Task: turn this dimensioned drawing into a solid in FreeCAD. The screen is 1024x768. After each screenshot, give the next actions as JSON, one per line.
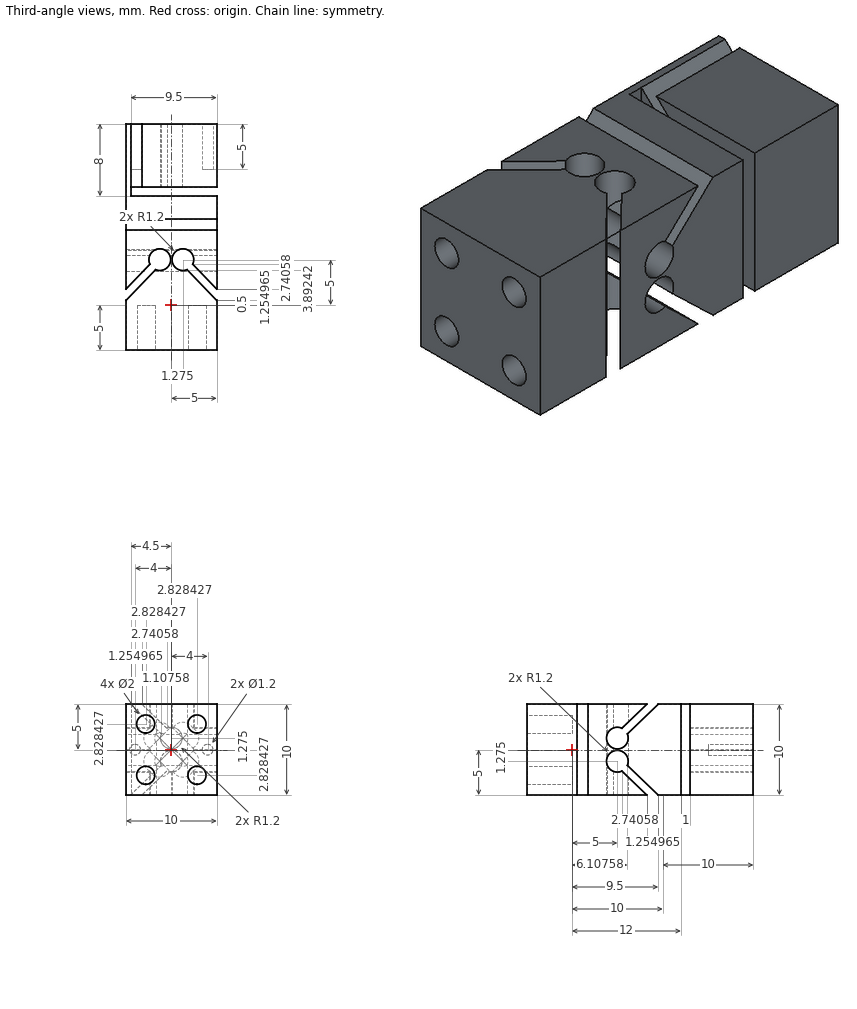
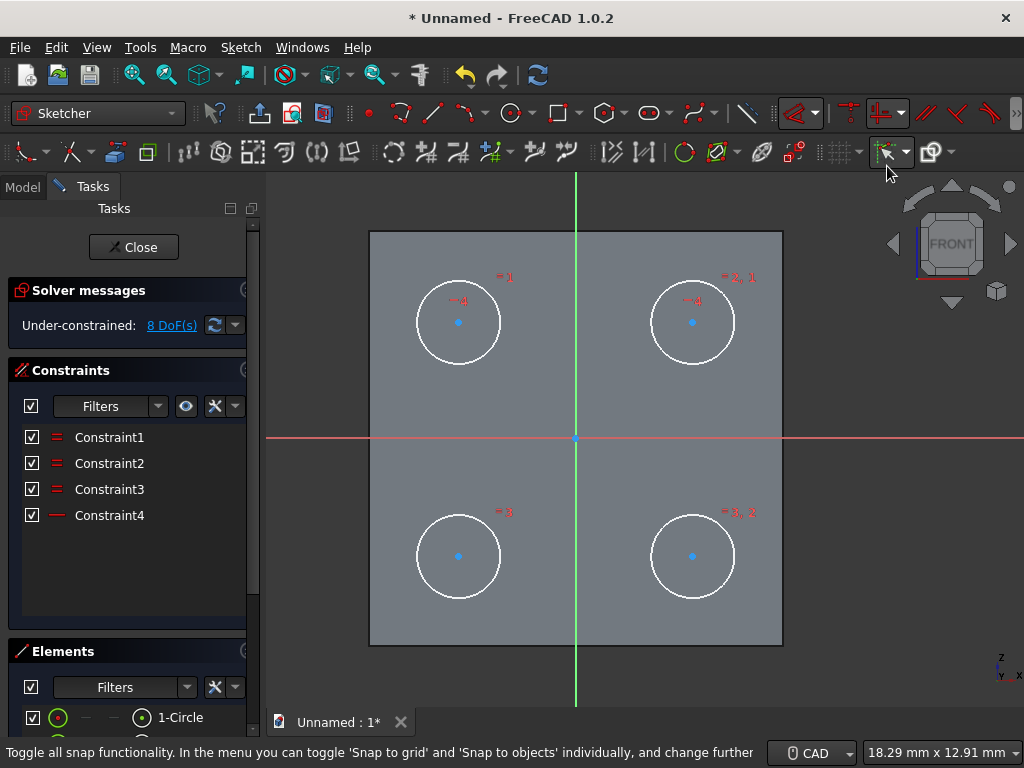
{"action": "left_click", "coordinate": [693, 322]}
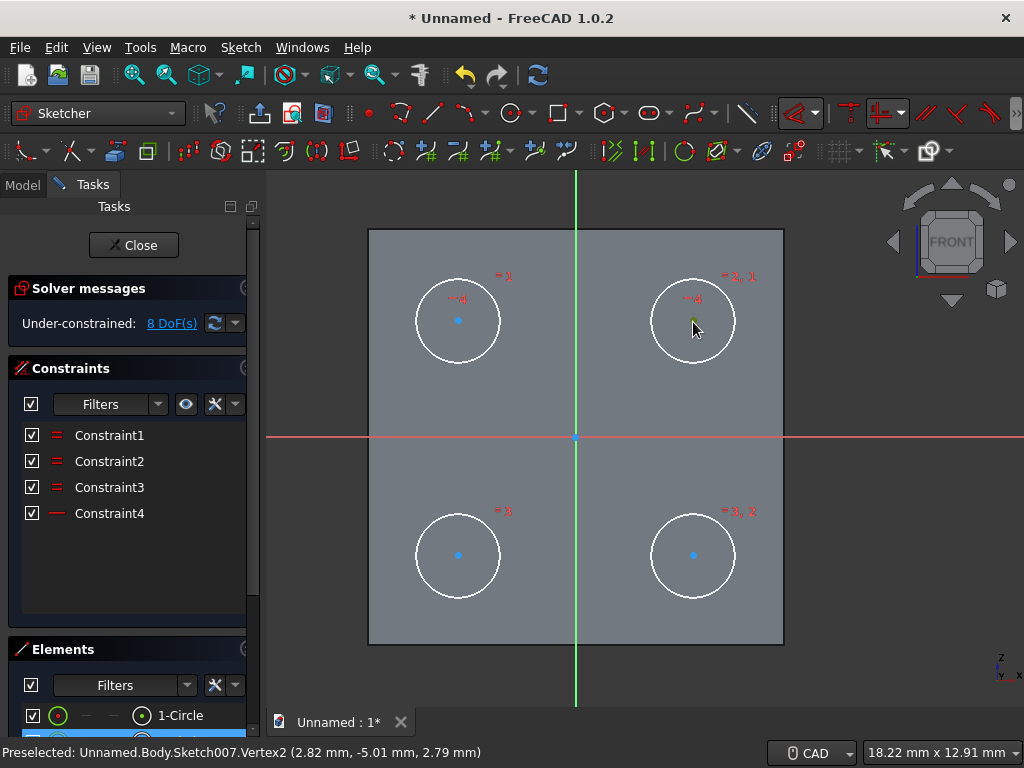
{"action": "left_click", "coordinate": [693, 556]}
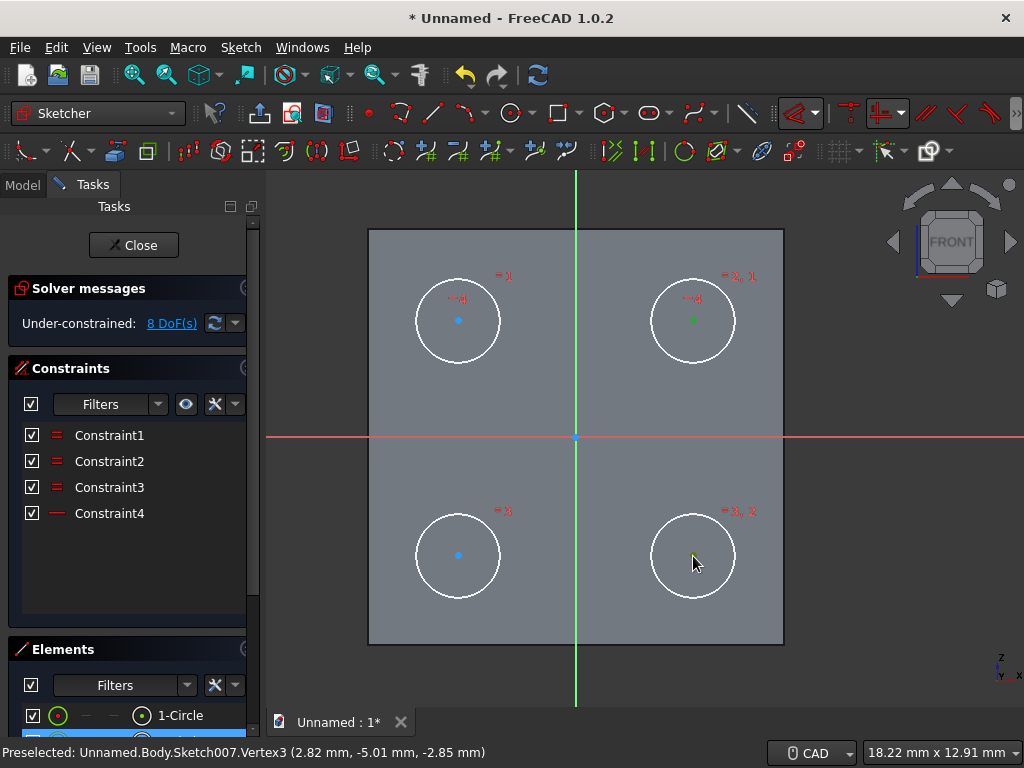
{"action": "left_click", "coordinate": [904, 114]}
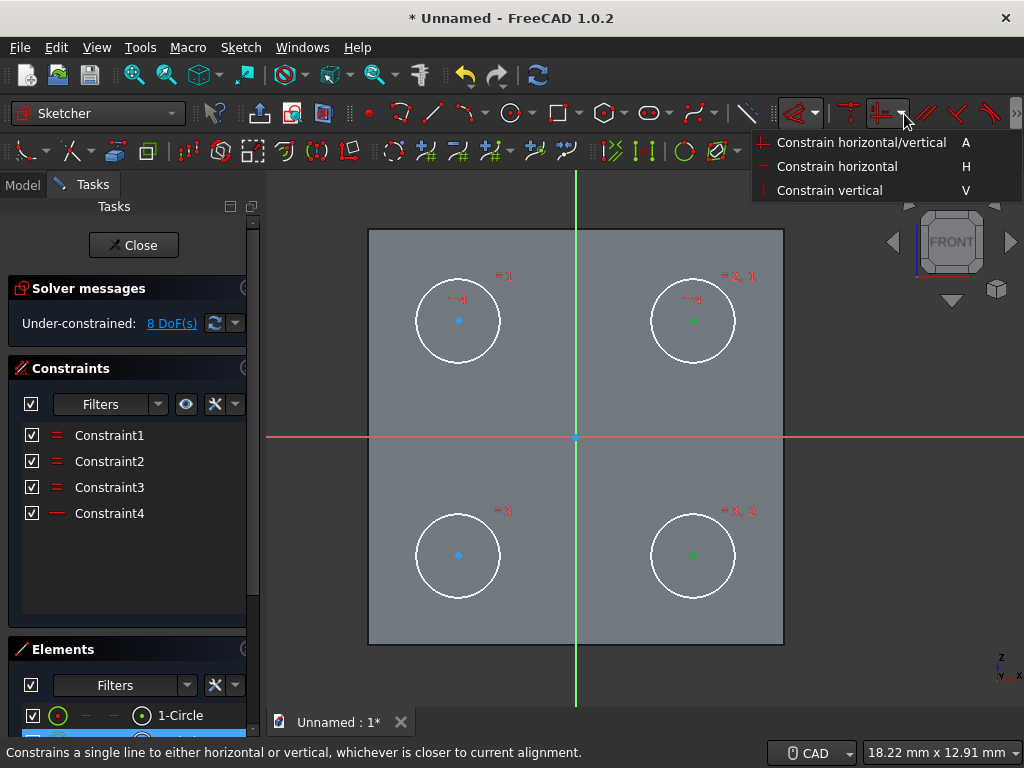
{"action": "left_click", "coordinate": [887, 190]}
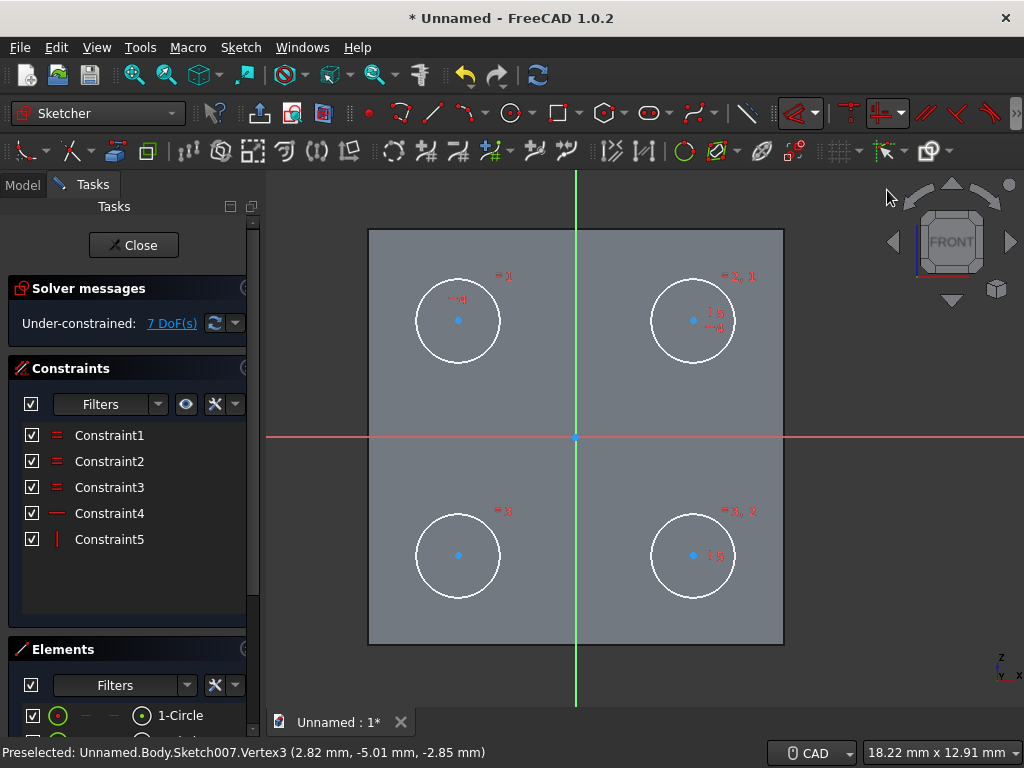
{"action": "left_click", "coordinate": [458, 321]}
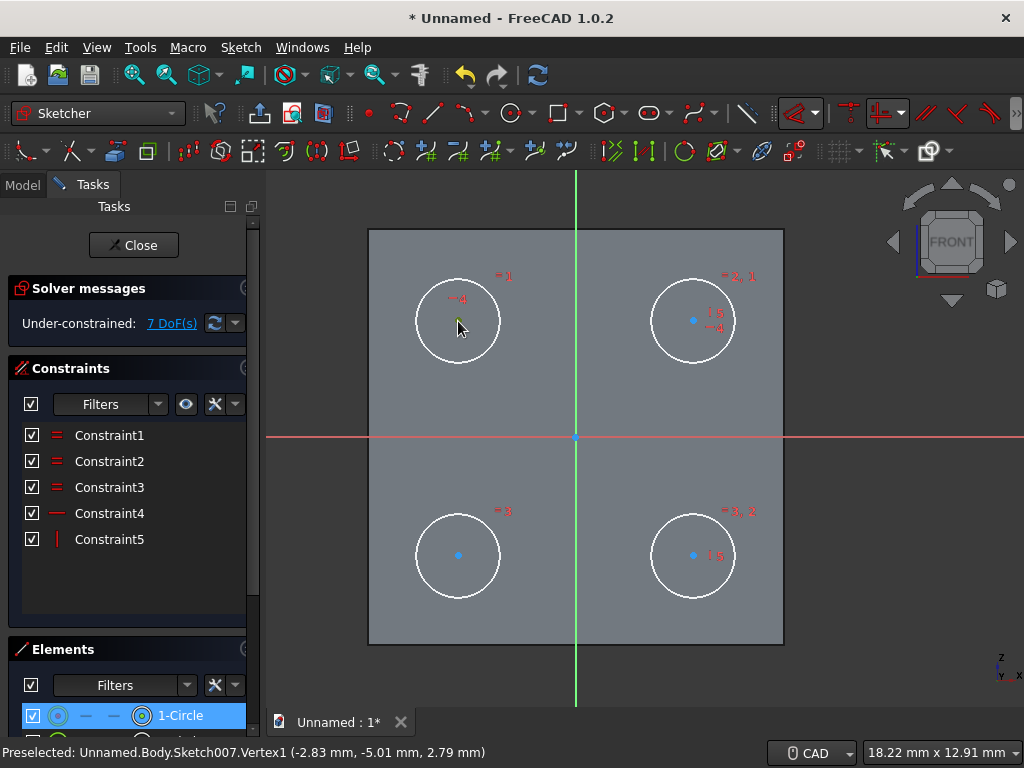
{"action": "left_click", "coordinate": [458, 556]}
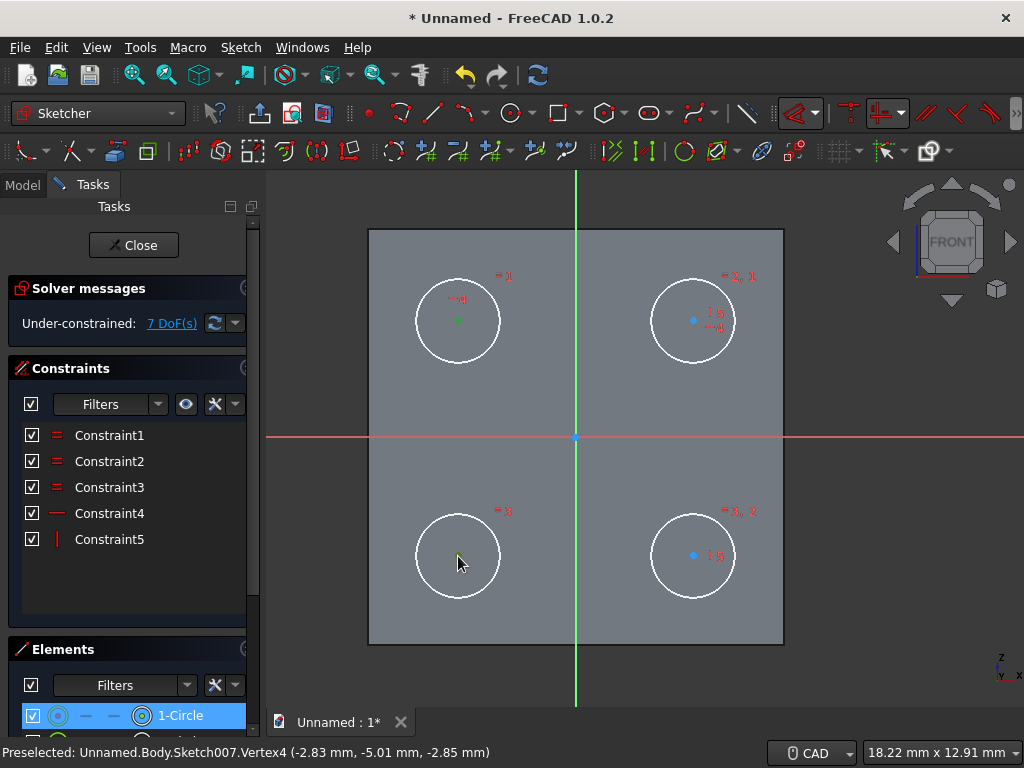
{"action": "left_click", "coordinate": [904, 114]}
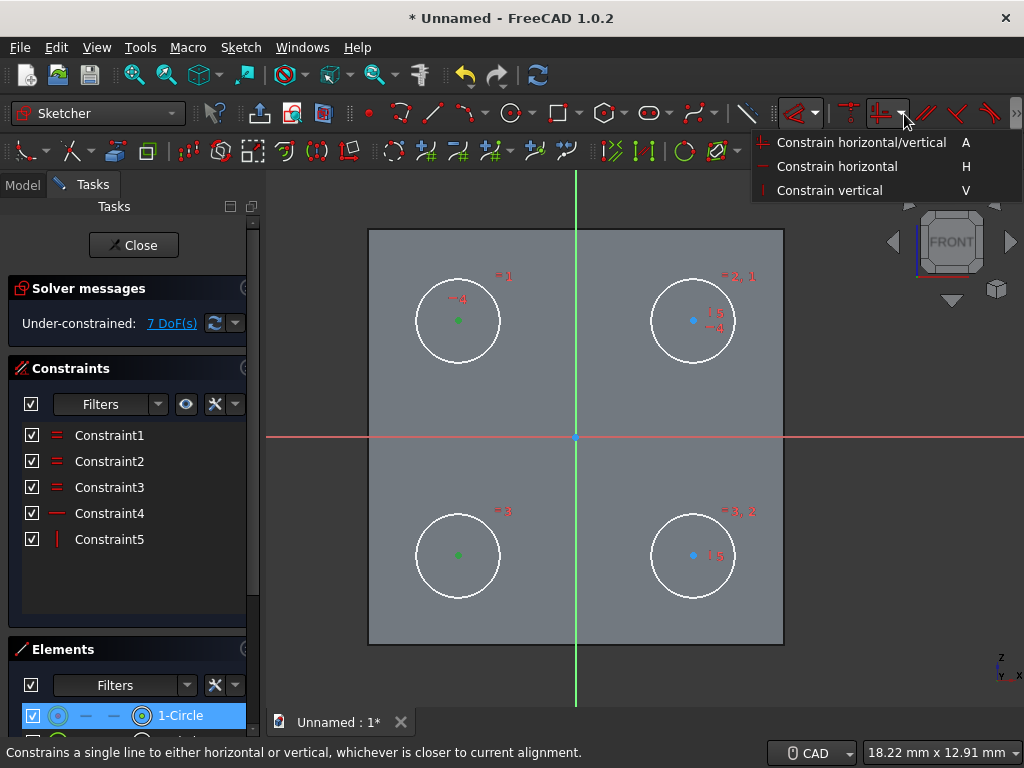
{"action": "left_click", "coordinate": [887, 190]}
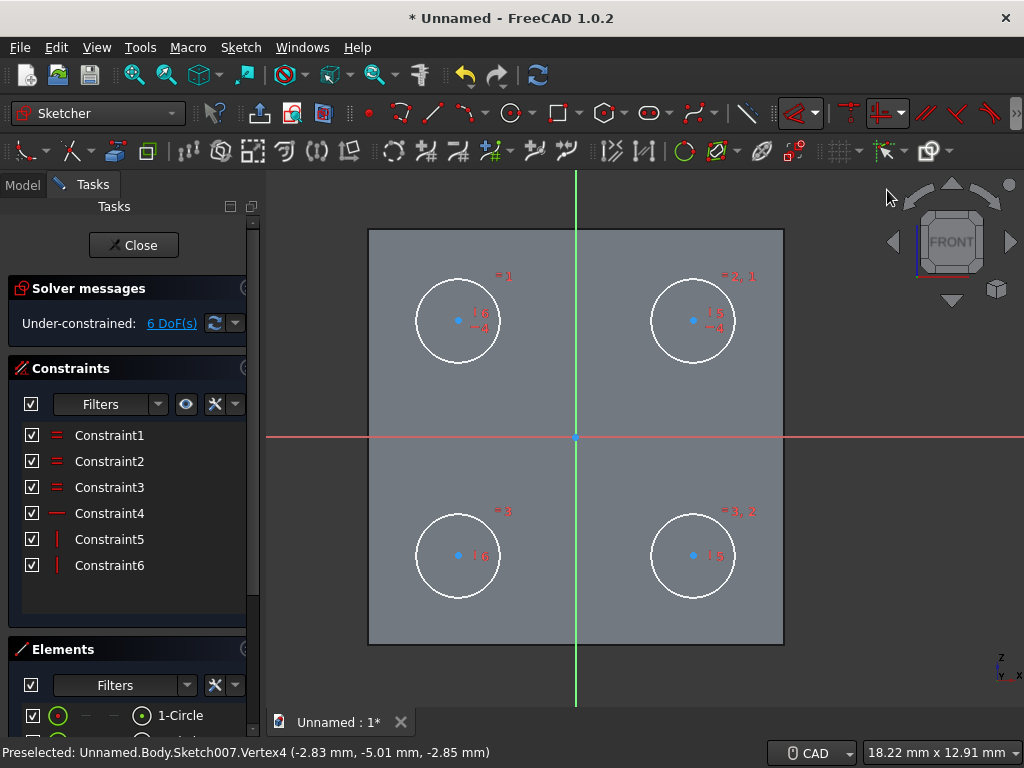
{"action": "left_click", "coordinate": [693, 556]}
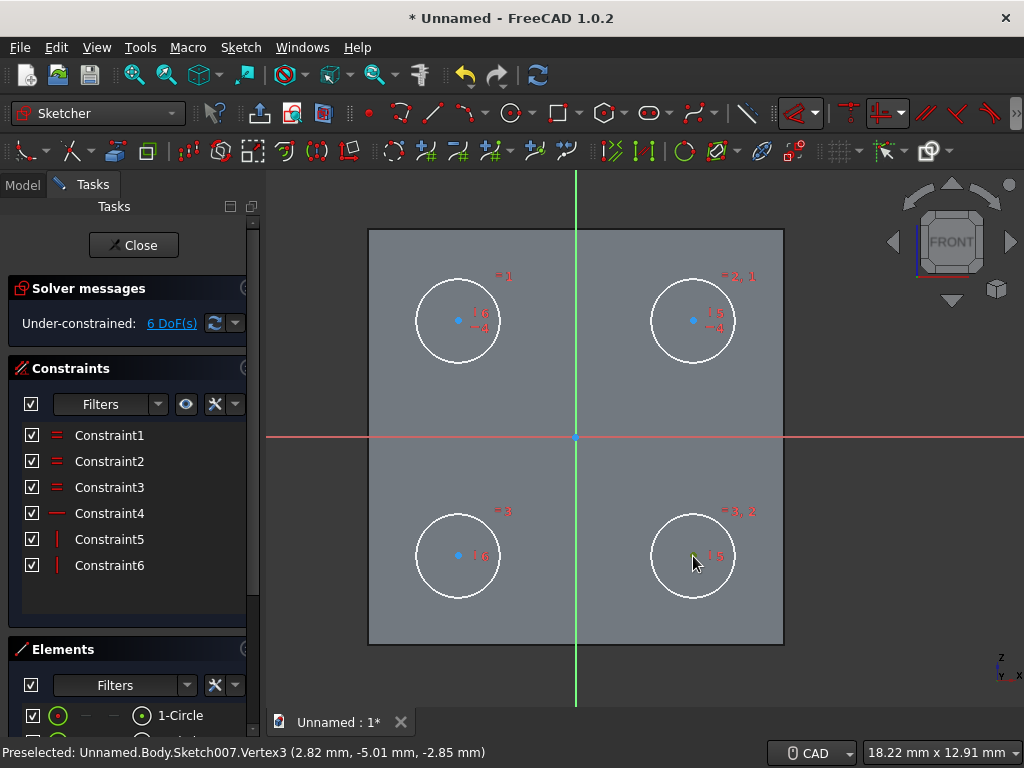
{"action": "left_click", "coordinate": [458, 556]}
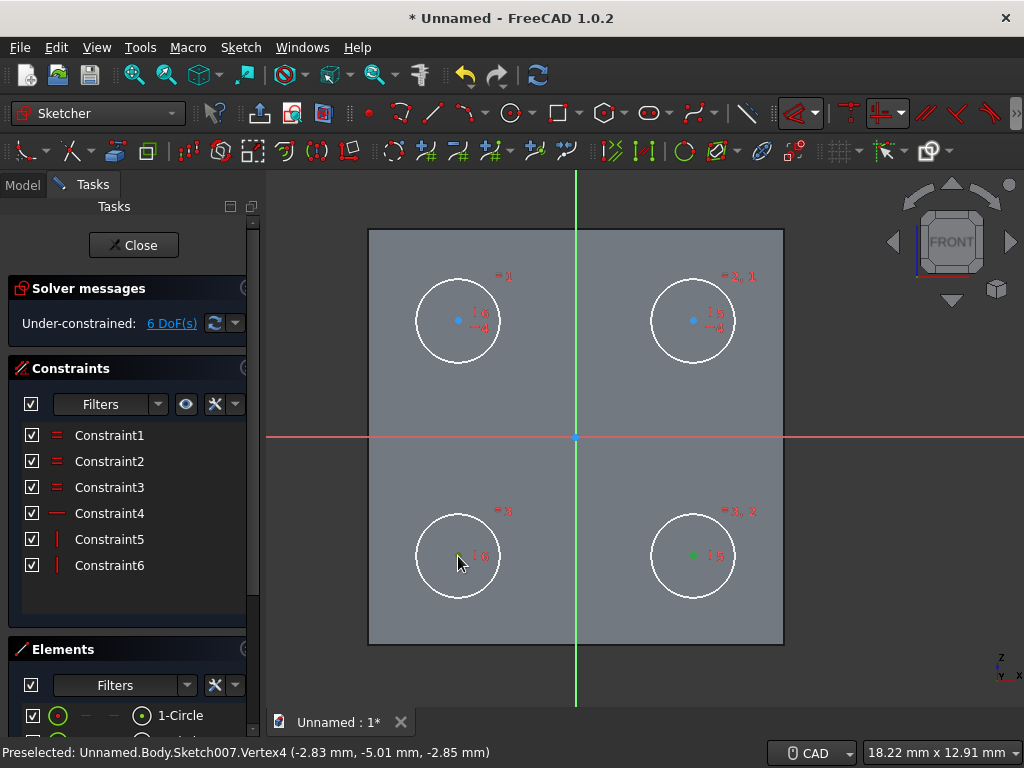
{"action": "key", "text": "h"}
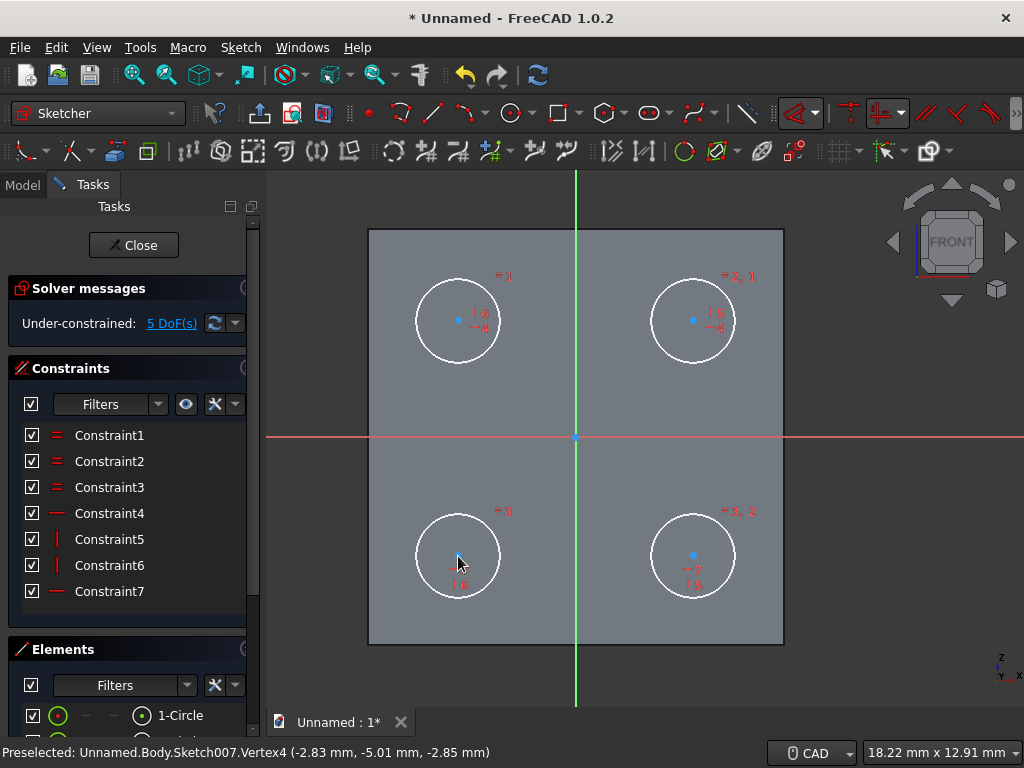
{"action": "left_click", "coordinate": [487, 291]}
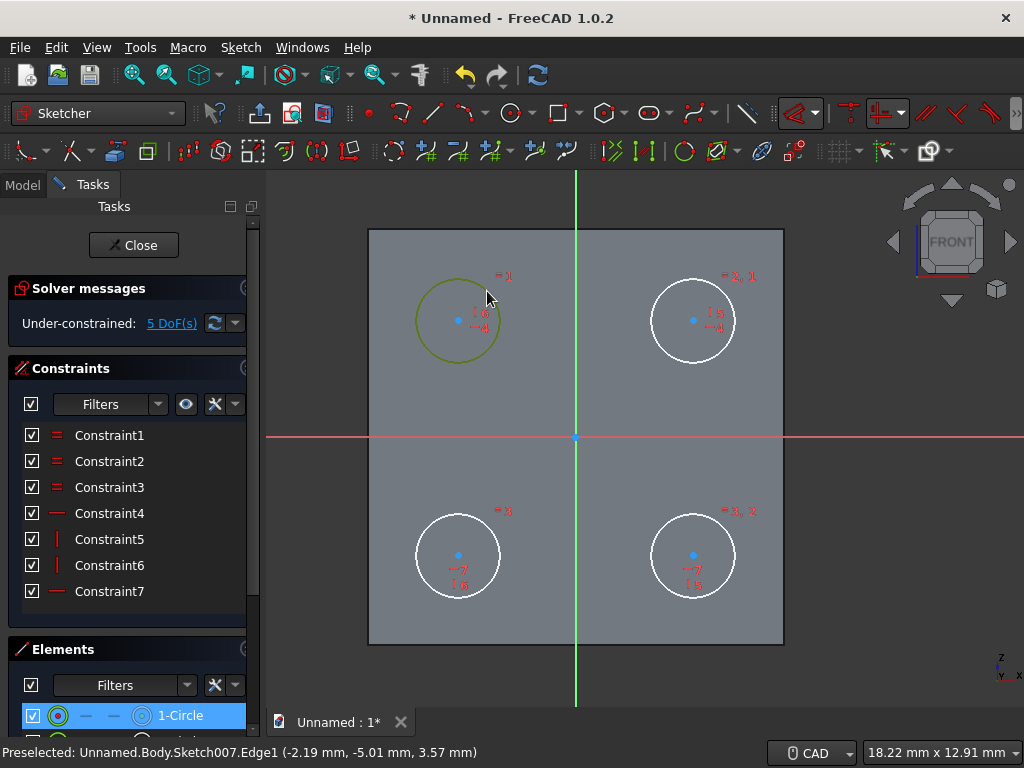
{"action": "key", "text": "k o"}